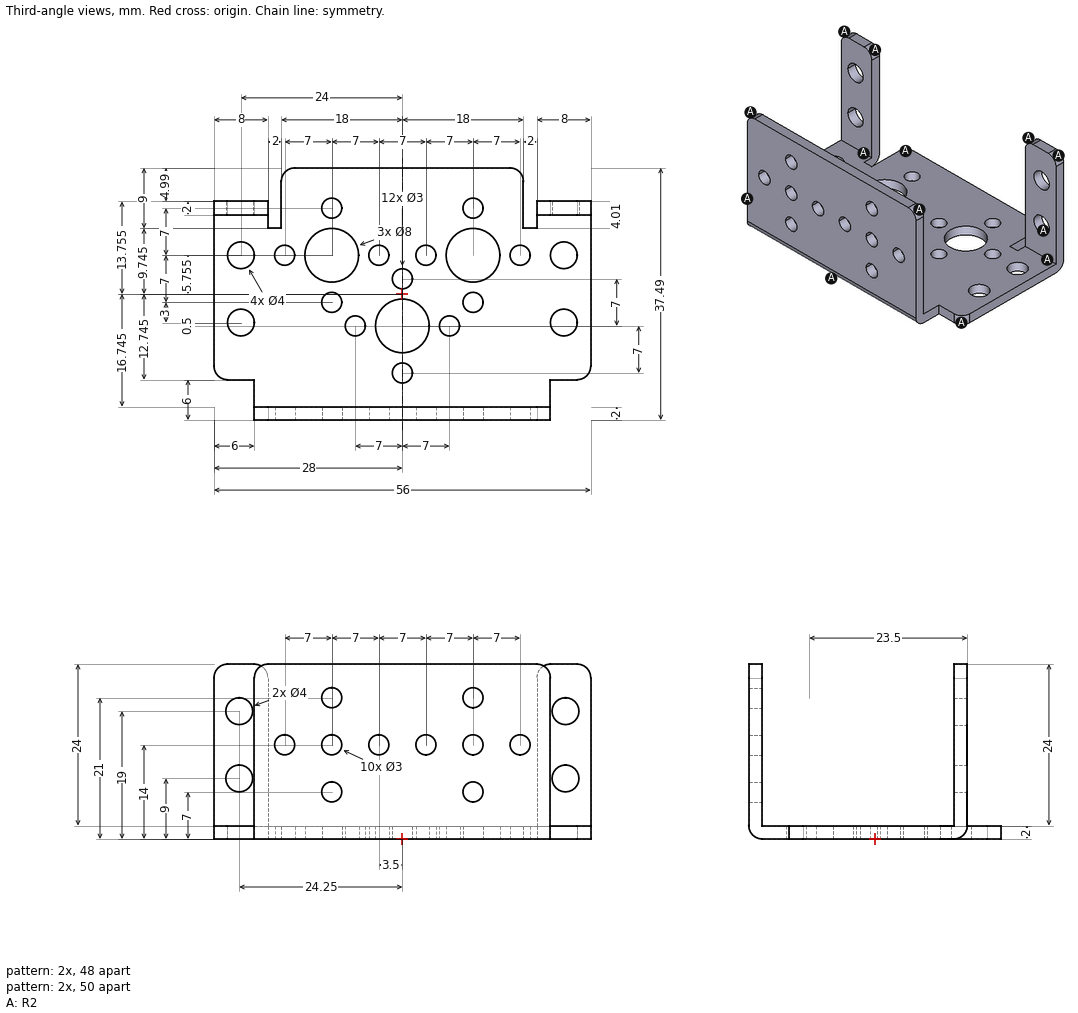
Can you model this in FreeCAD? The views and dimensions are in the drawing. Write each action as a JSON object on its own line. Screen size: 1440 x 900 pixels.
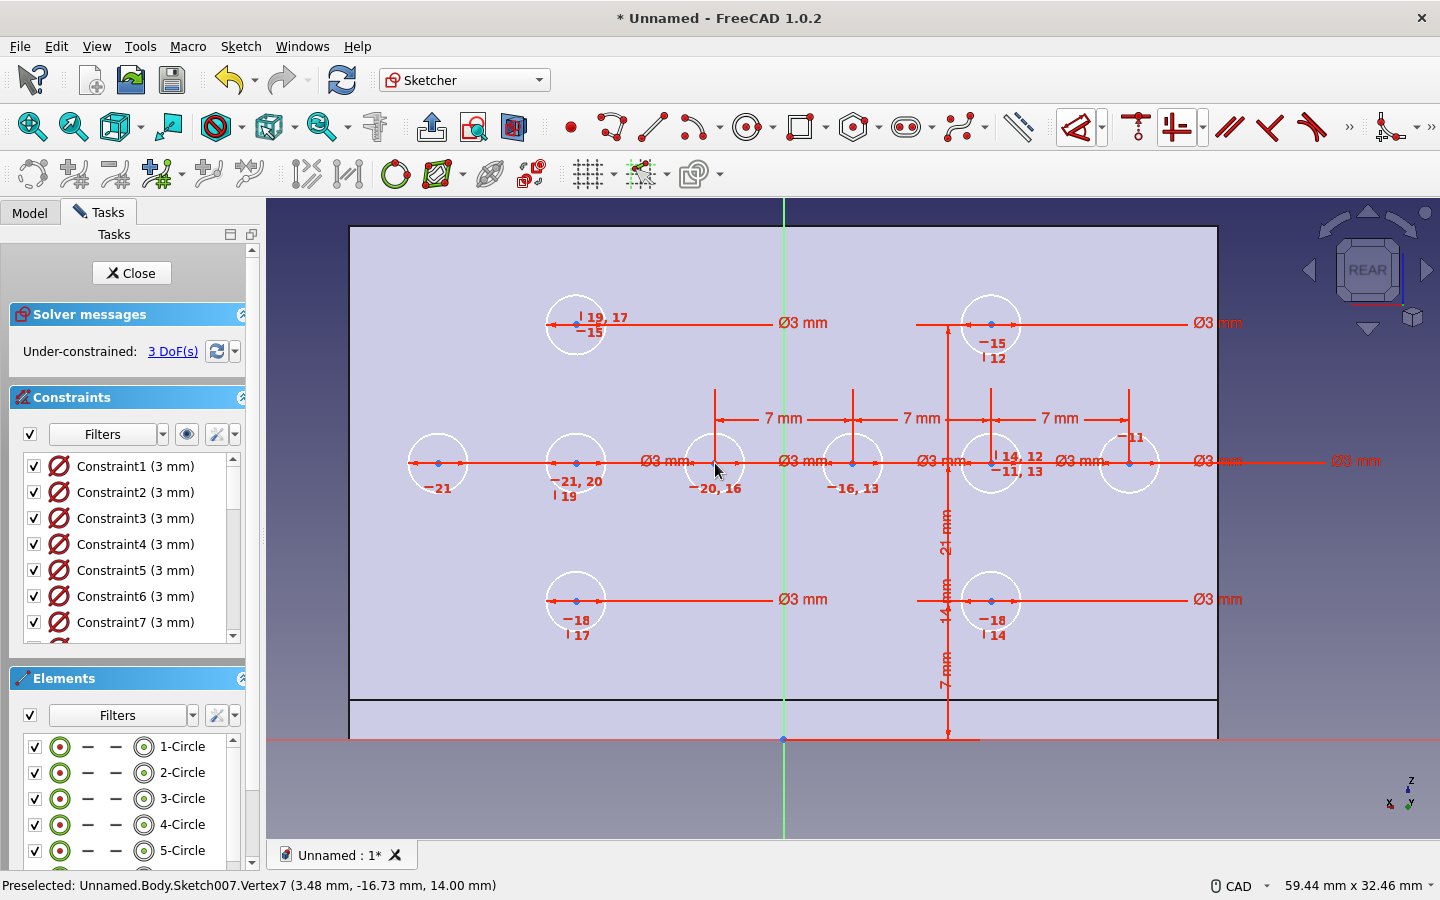
{"action": "left_click", "coordinate": [576, 325]}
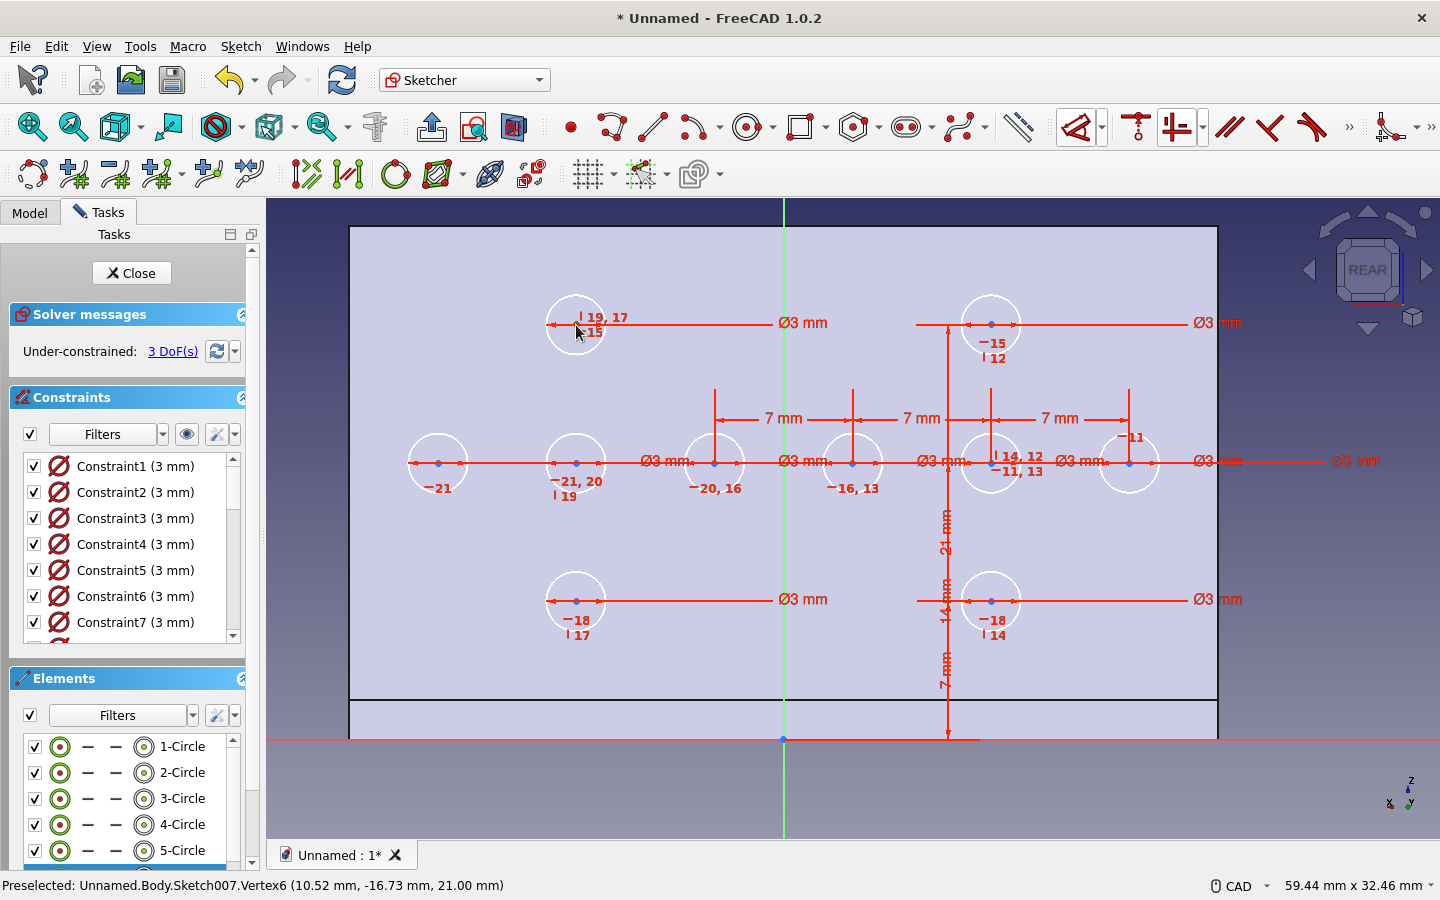
{"action": "left_click", "coordinate": [715, 463]}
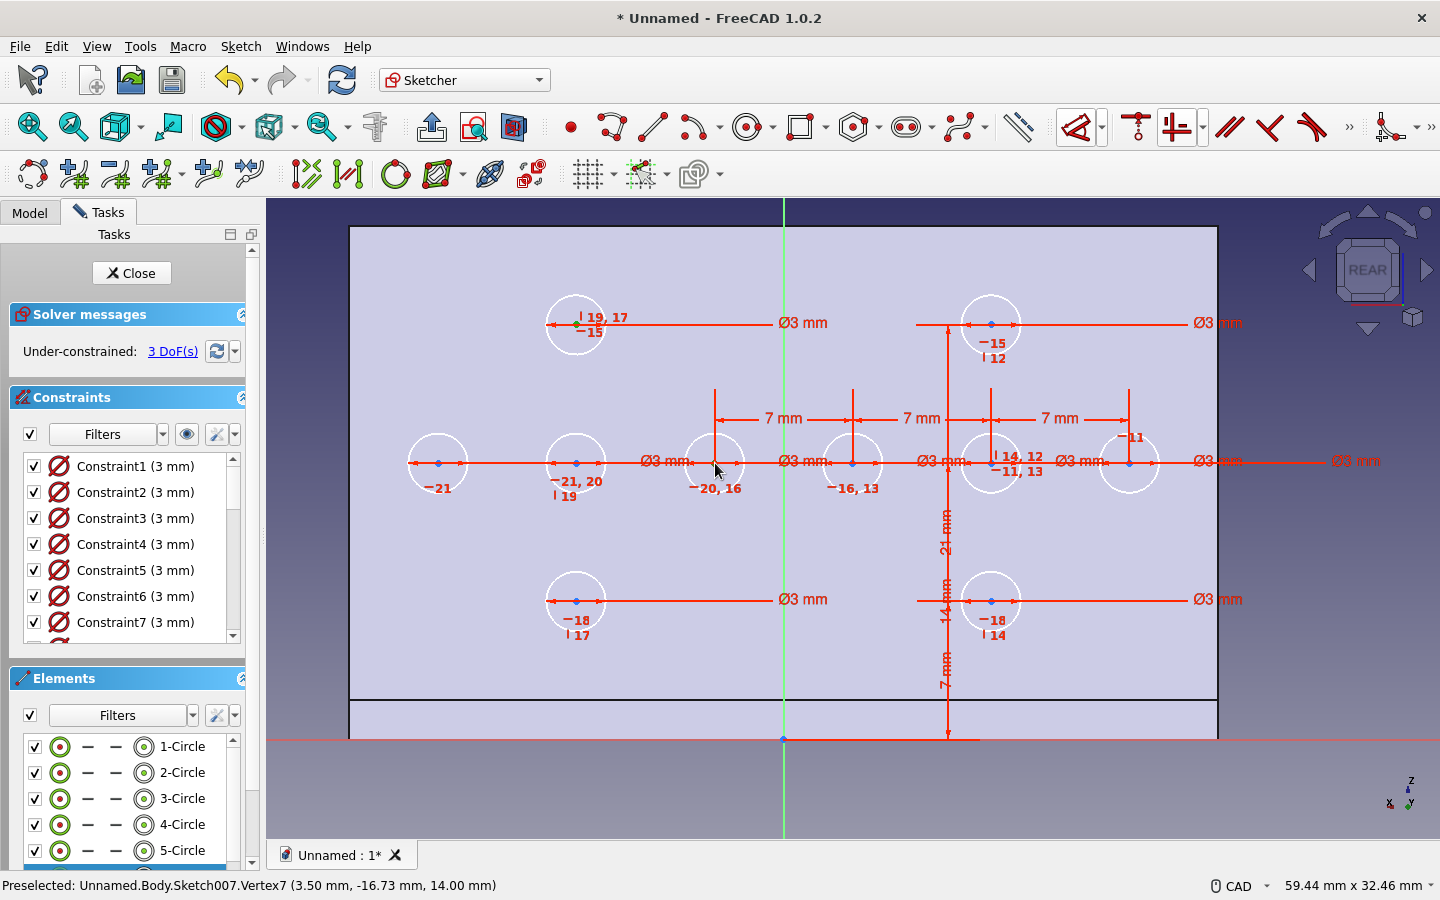
{"action": "key", "text": "l"}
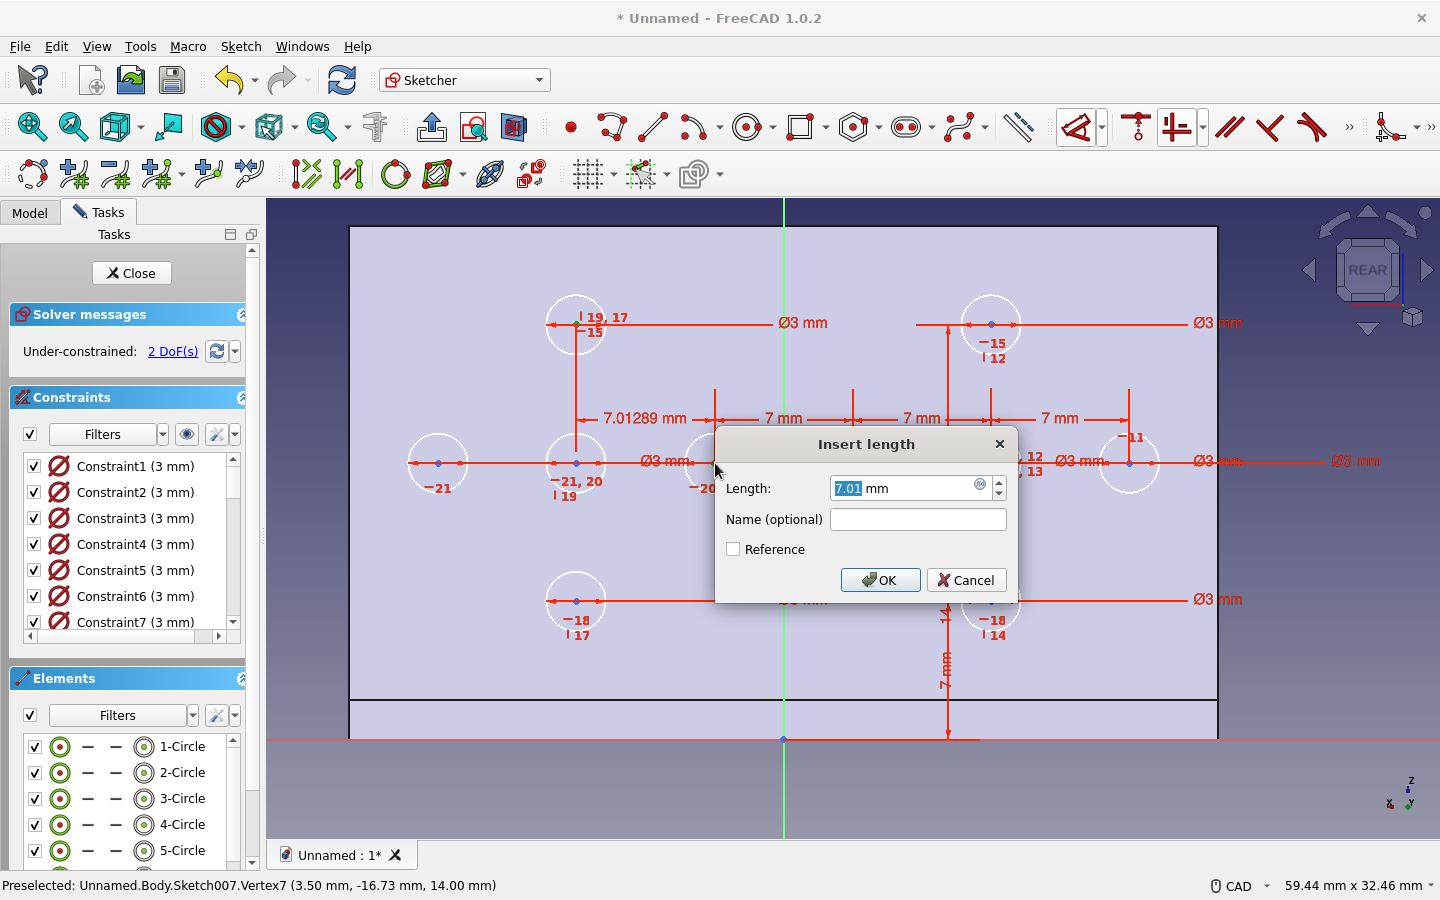
{"action": "type", "text": "7"}
{"action": "key", "text": "Return"}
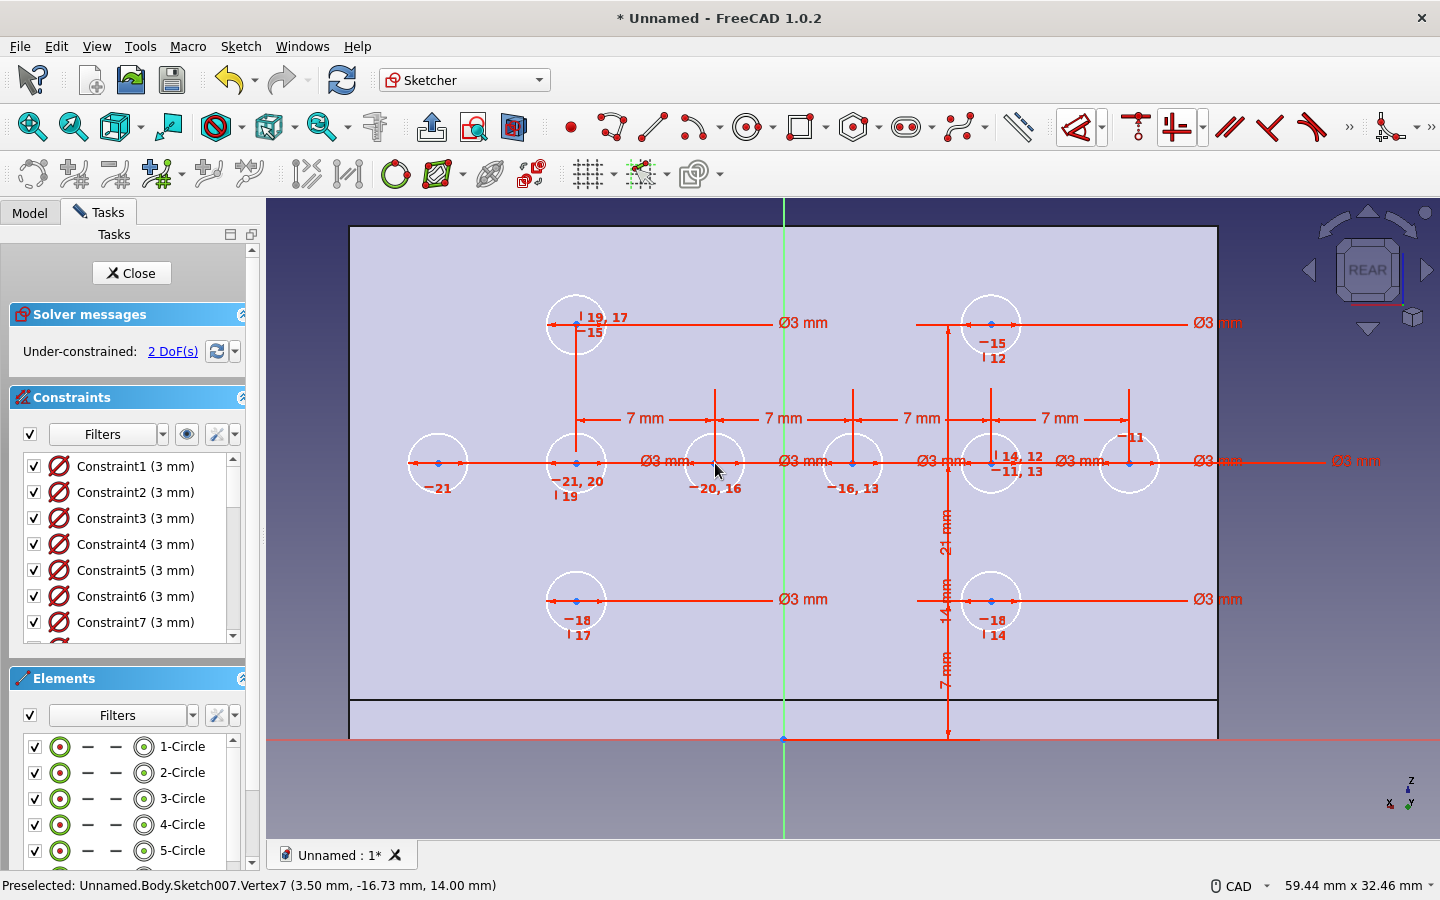
{"action": "left_click", "coordinate": [576, 463]}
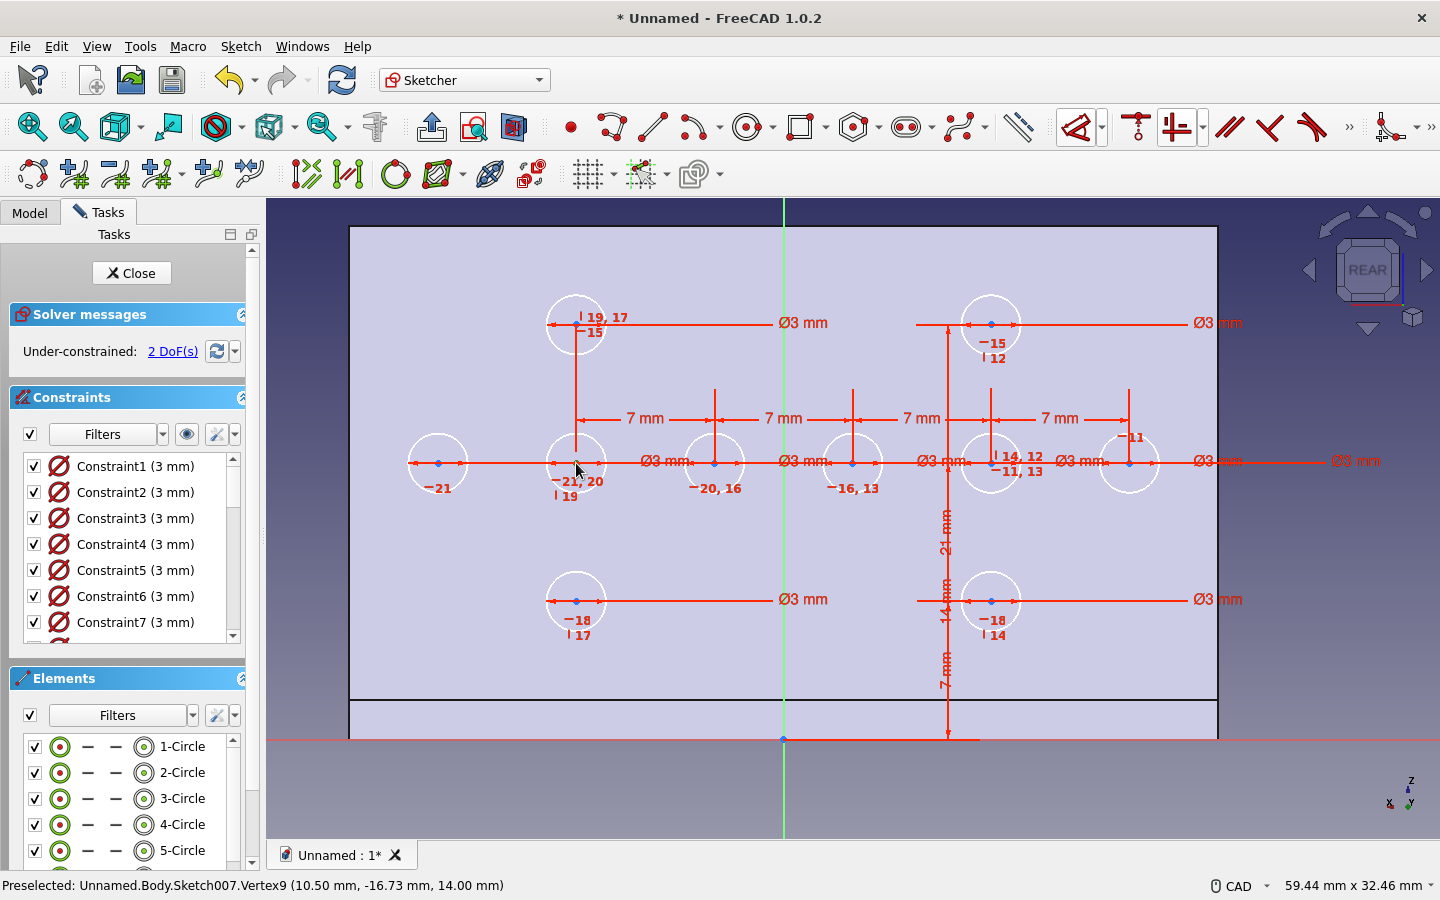
{"action": "left_click", "coordinate": [438, 463]}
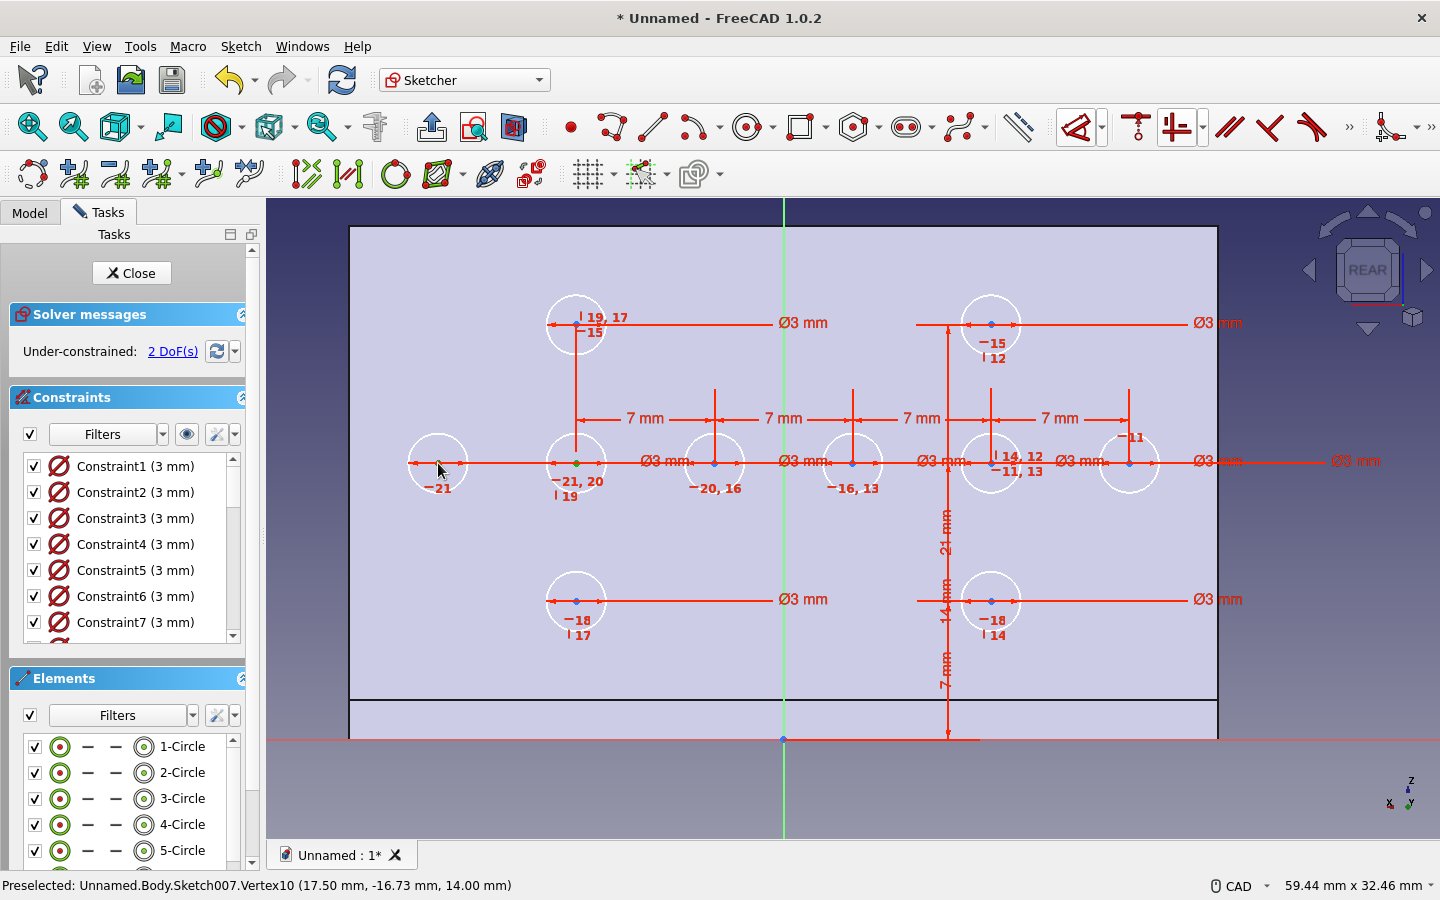
{"action": "key", "text": "l"}